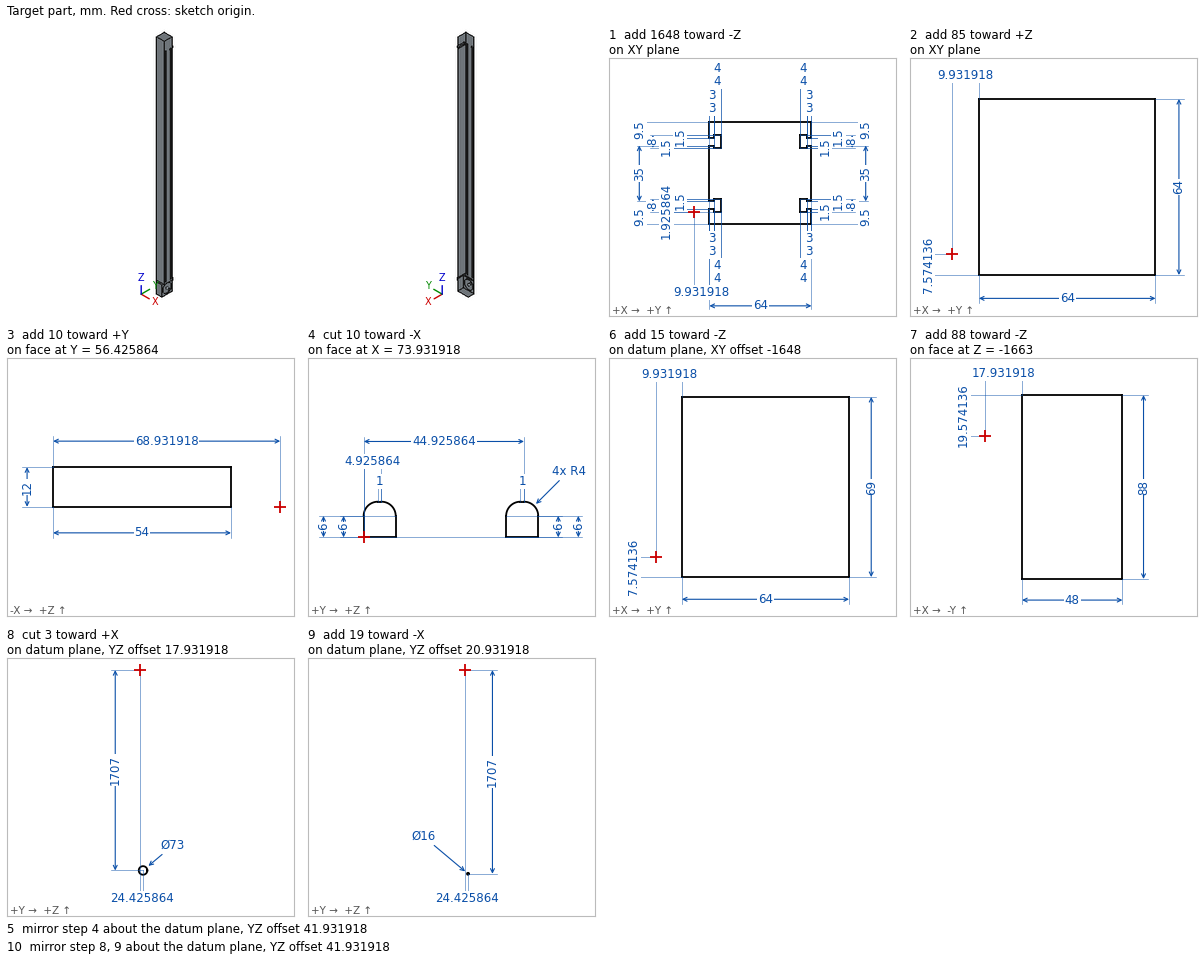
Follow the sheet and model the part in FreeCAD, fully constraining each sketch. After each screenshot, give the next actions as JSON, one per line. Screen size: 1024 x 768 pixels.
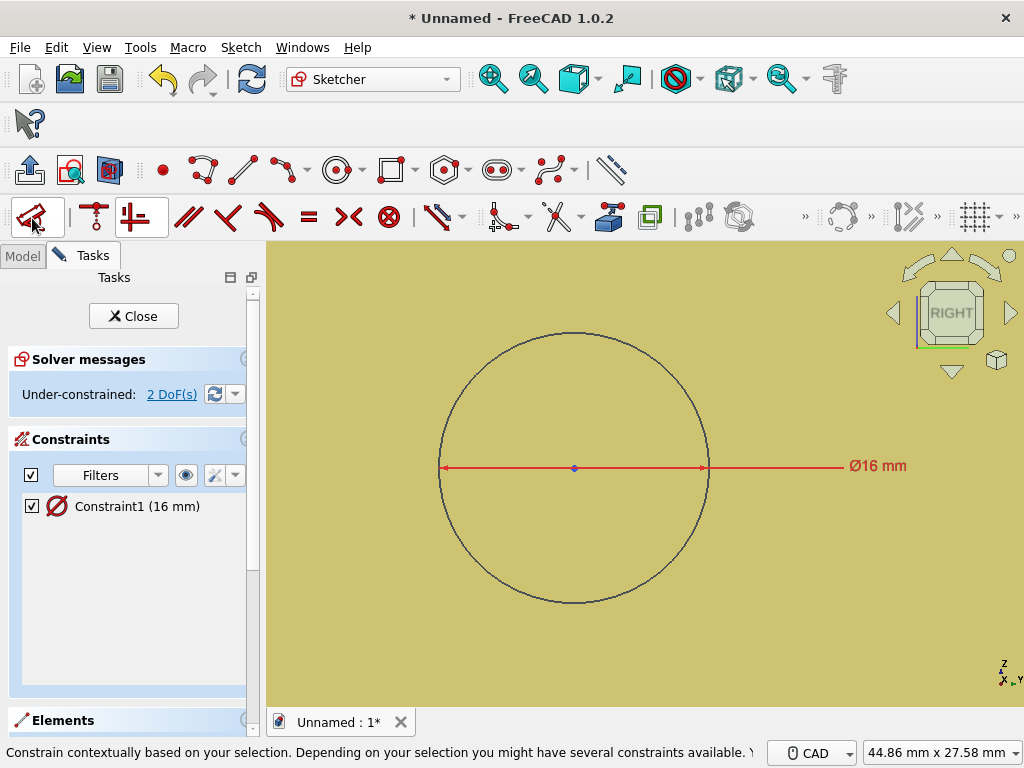
{"action": "left_click", "coordinate": [574, 468]}
{"action": "left_click", "coordinate": [608, 369]}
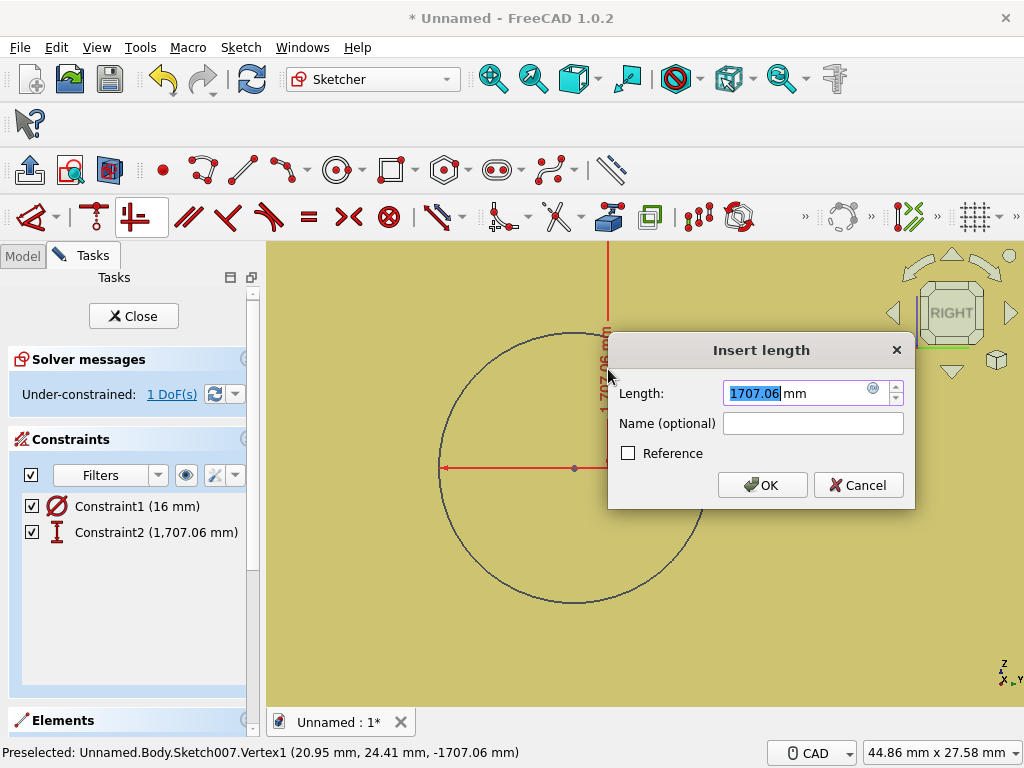
{"action": "type", "text": "1707"}
{"action": "key", "text": "Return"}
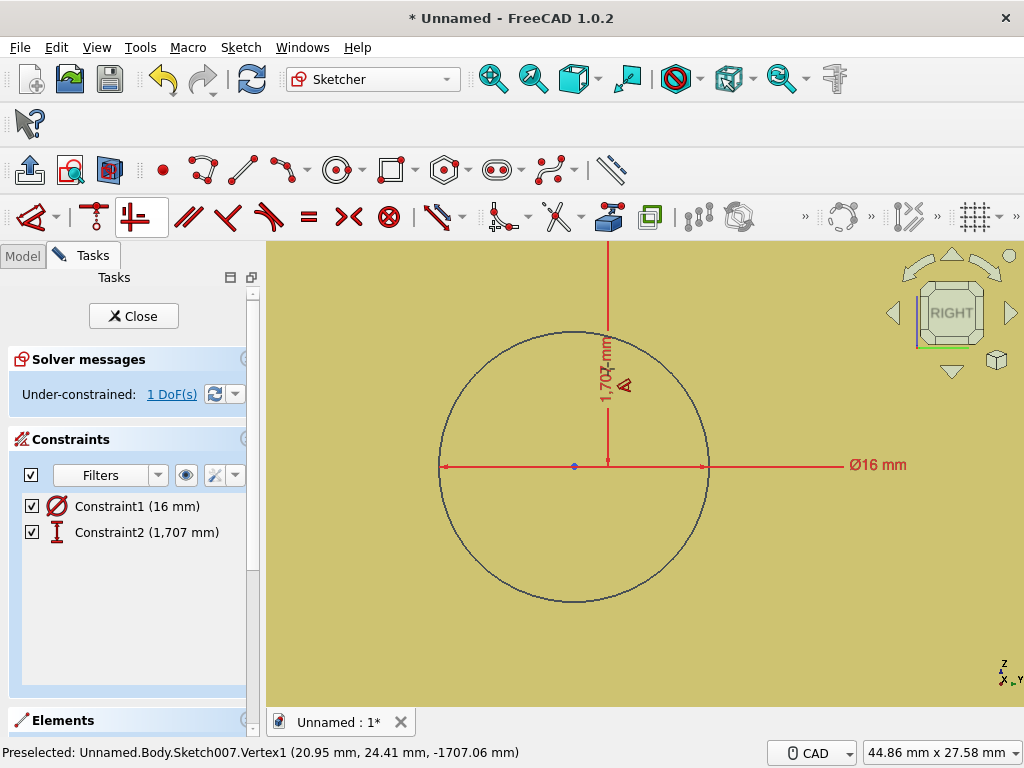
{"action": "left_click", "coordinate": [574, 467]}
{"action": "left_click", "coordinate": [370, 501]}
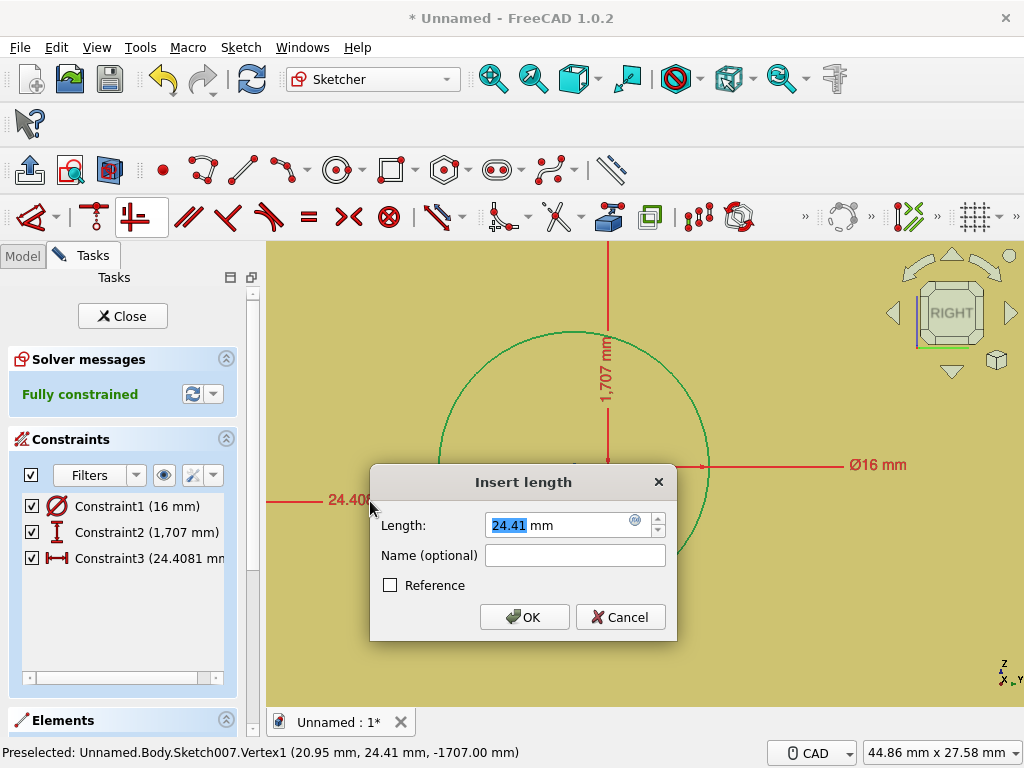
{"action": "type", "text": "24.425864"}
{"action": "key", "text": "Return"}
{"action": "key", "text": "Escape"}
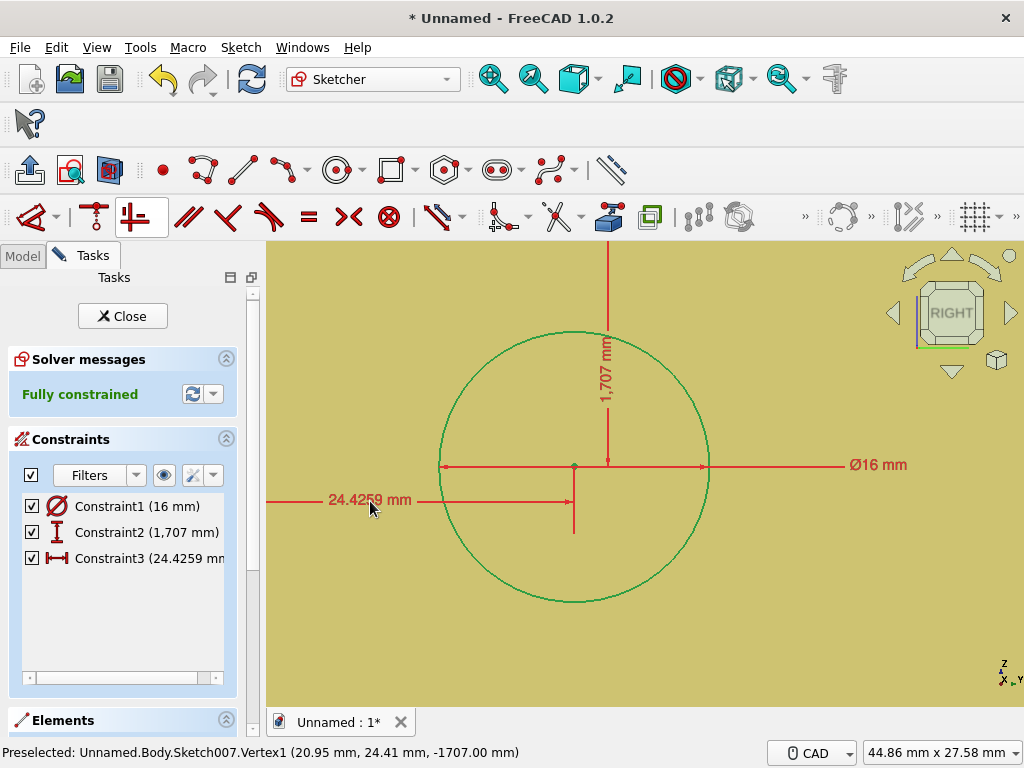
{"action": "left_click", "coordinate": [123, 316]}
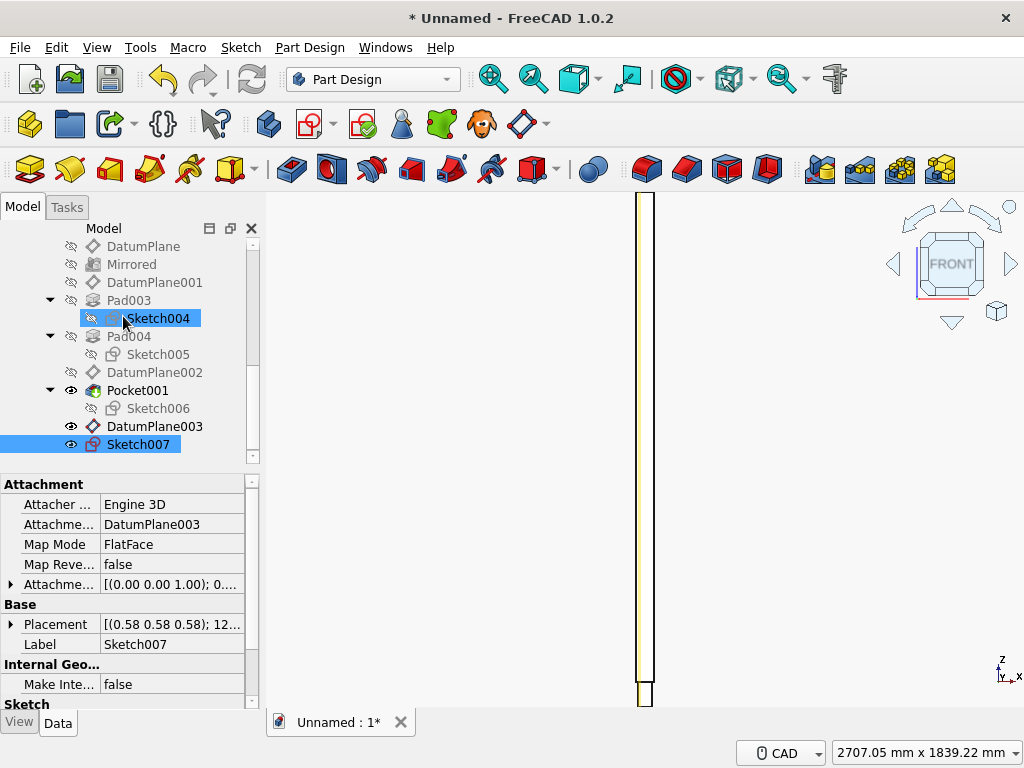
{"action": "left_click", "coordinate": [30, 170]}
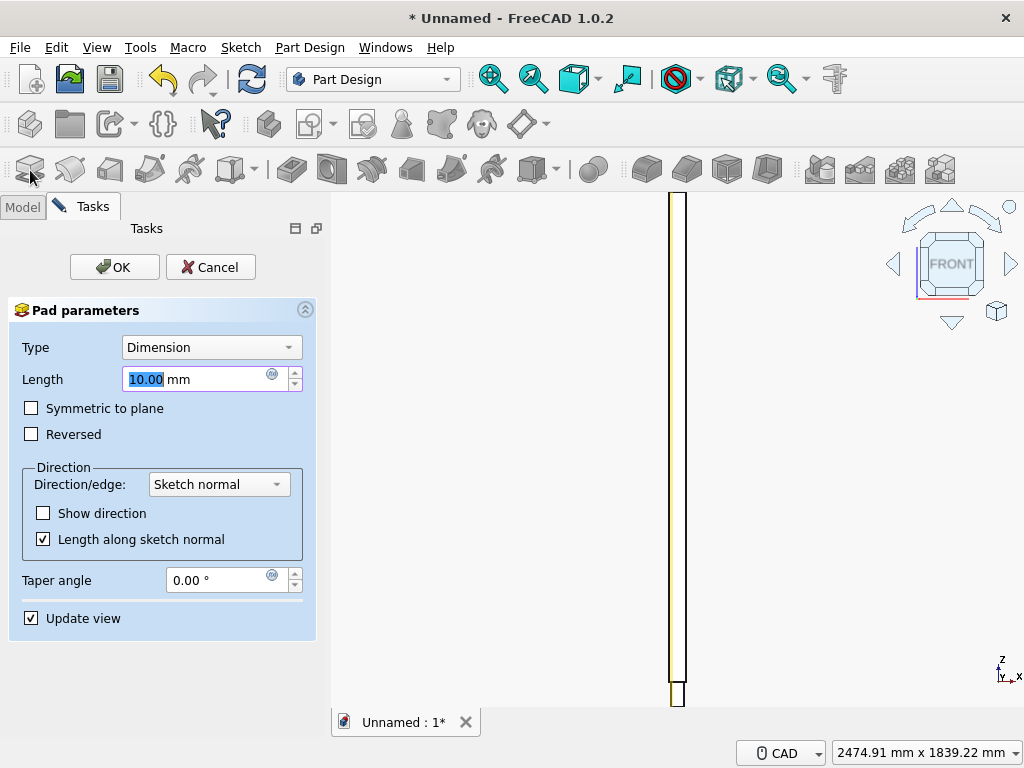
{"action": "type", "text": "19"}
{"action": "key", "text": "Tab"}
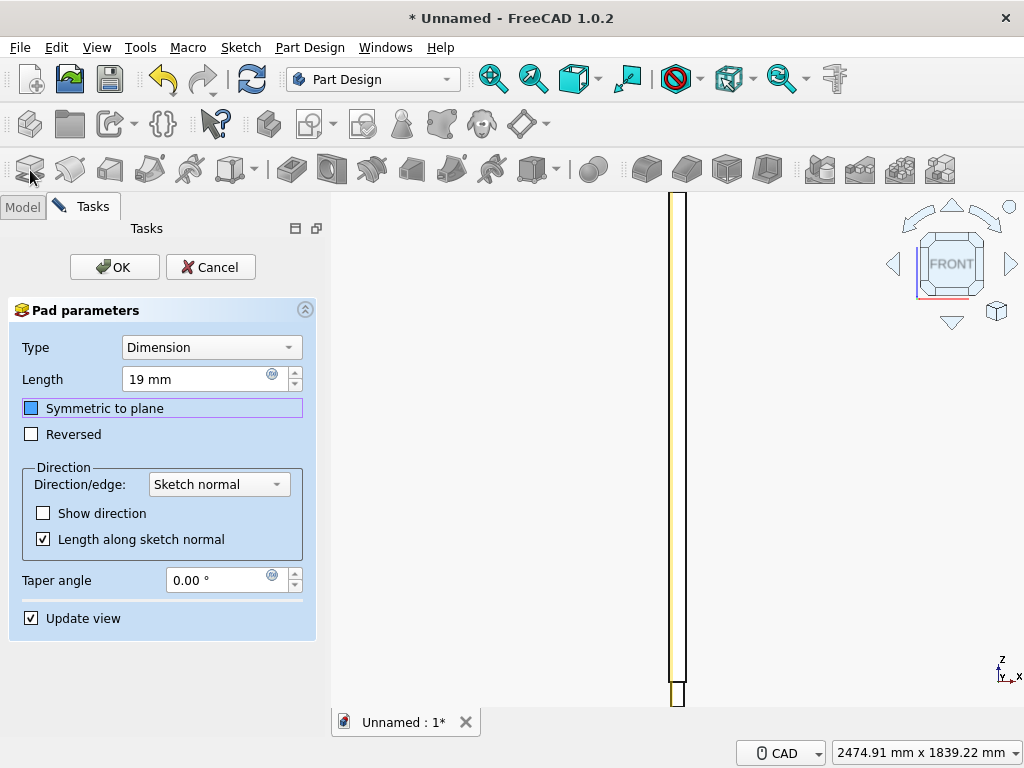
{"action": "left_click", "coordinate": [30, 434]}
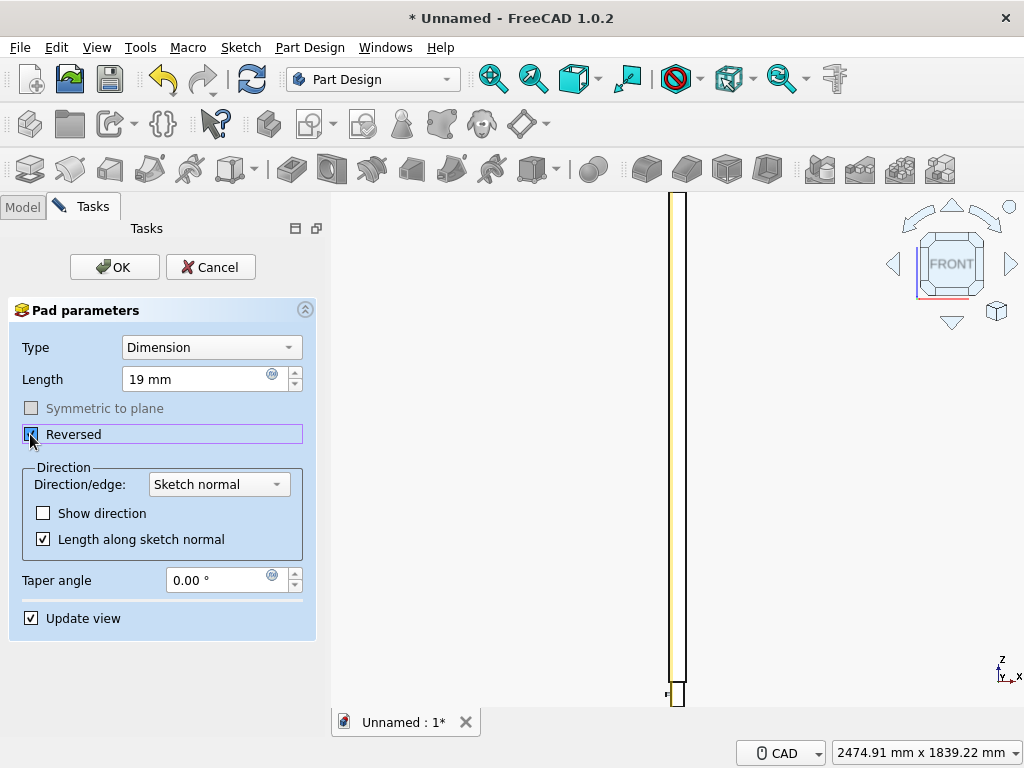
{"action": "left_click", "coordinate": [115, 267]}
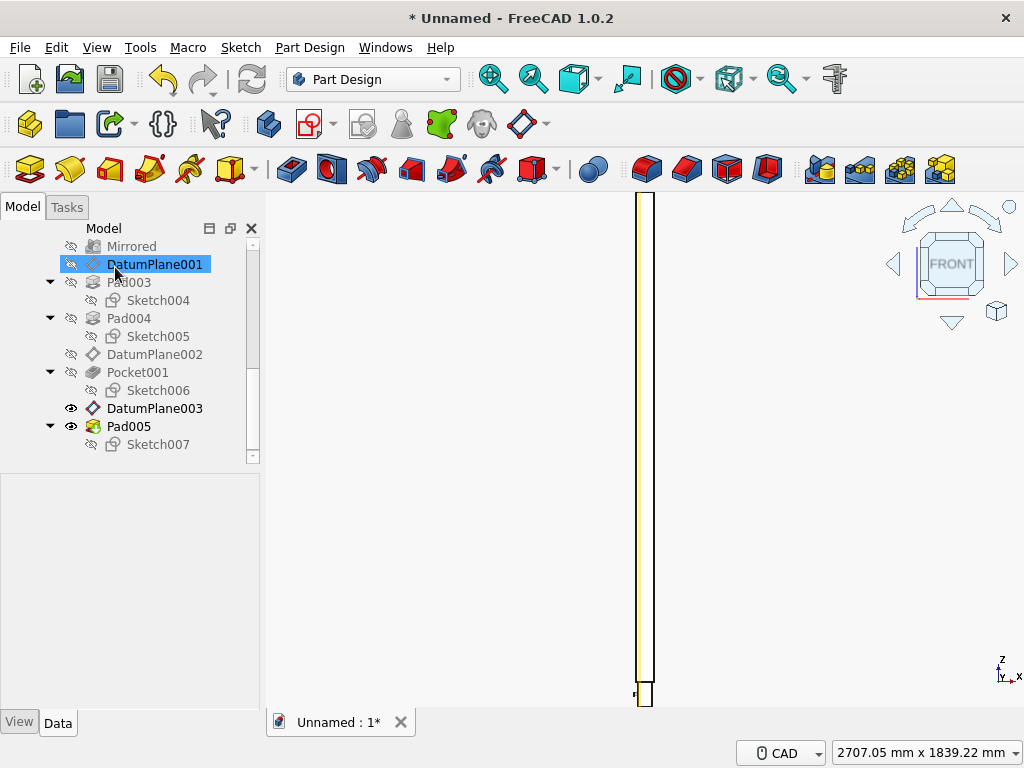
{"action": "left_click", "coordinate": [116, 408]}
{"action": "key", "text": "space"}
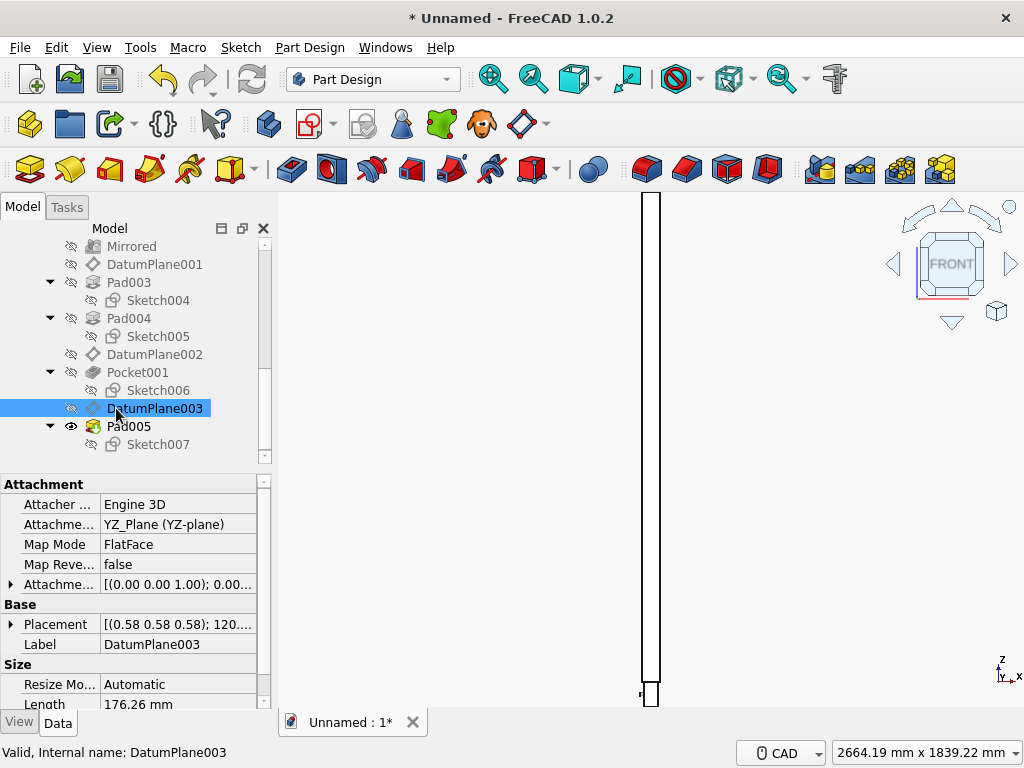
{"action": "left_click", "coordinate": [494, 80]}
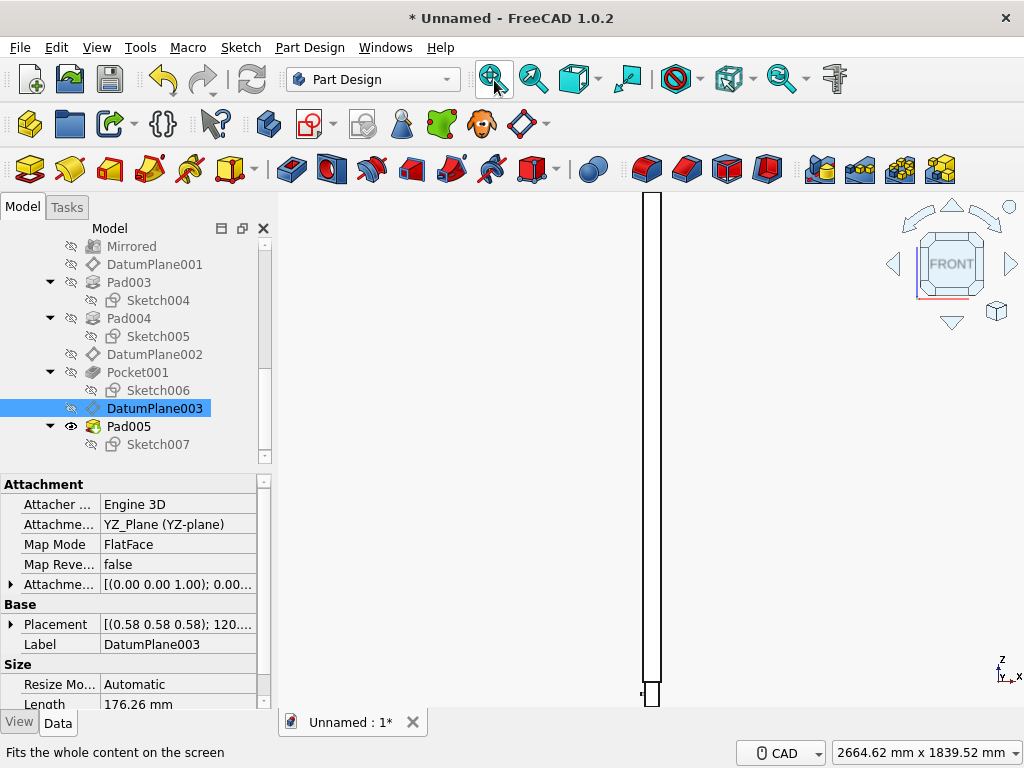
{"action": "scroll", "coordinate": [140, 350], "scroll_direction": "down", "scroll_amount": 3}